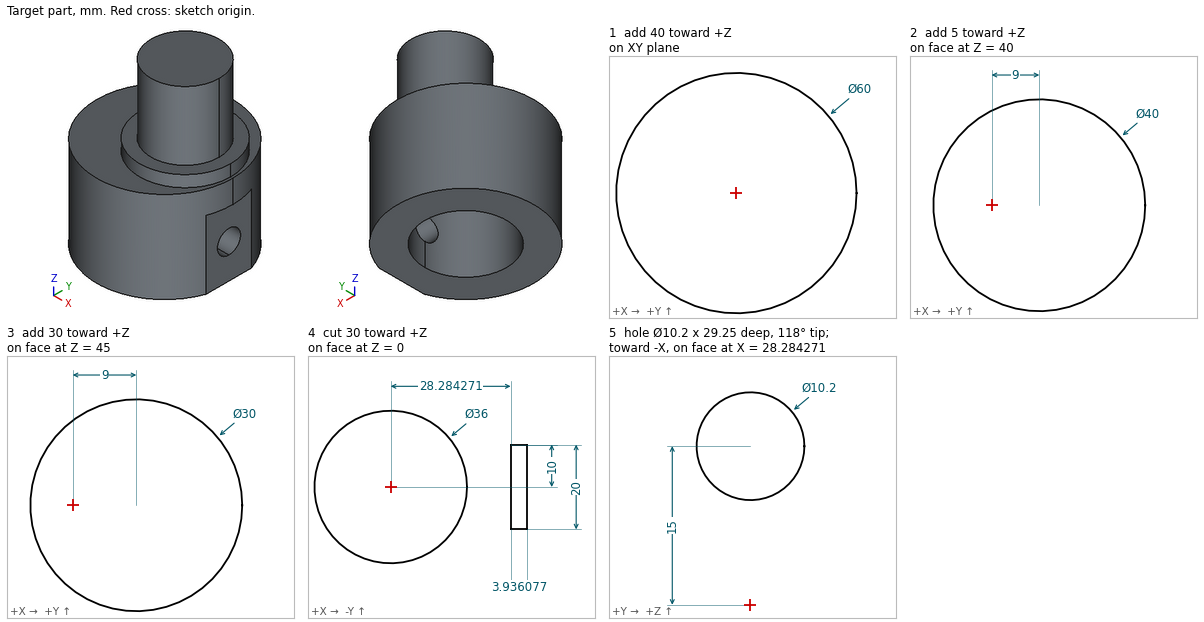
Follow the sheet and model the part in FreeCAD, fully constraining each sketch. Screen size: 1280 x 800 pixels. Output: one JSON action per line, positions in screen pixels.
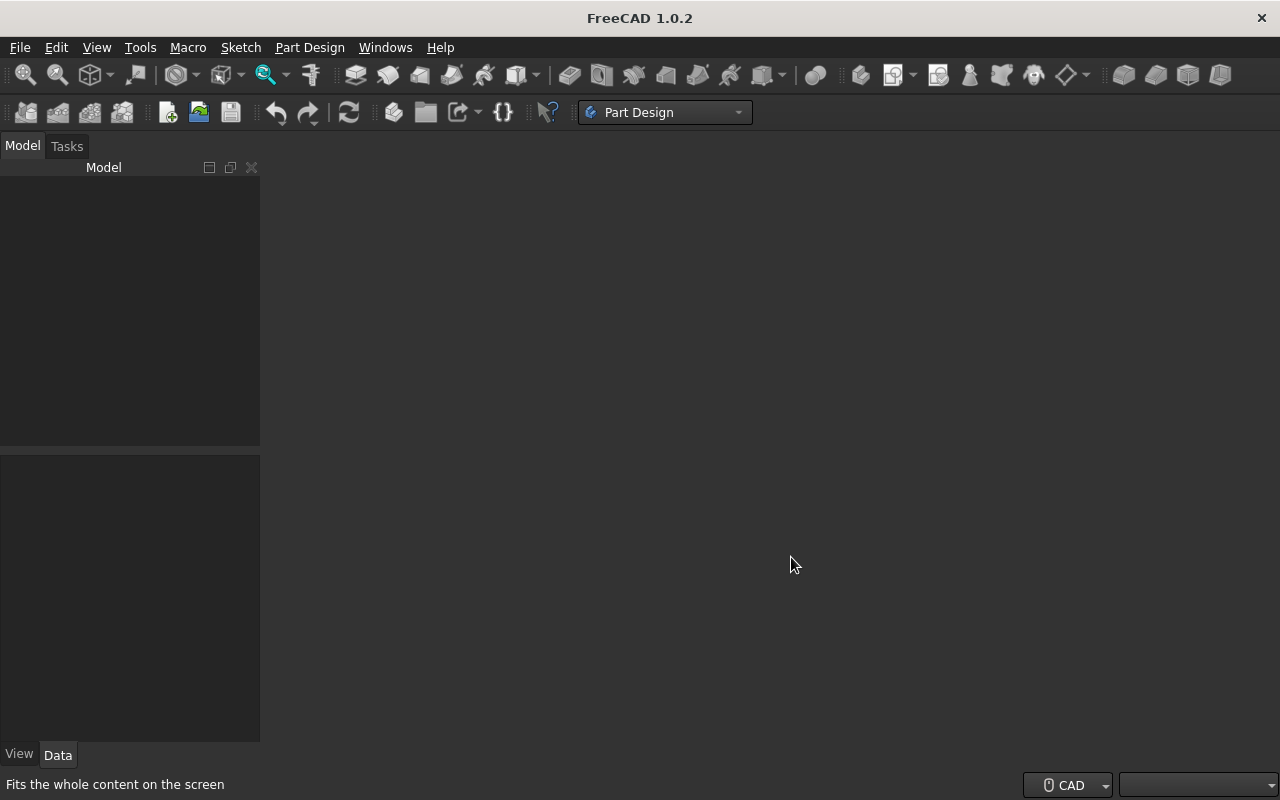
{"action": "key", "text": "ctrl+n"}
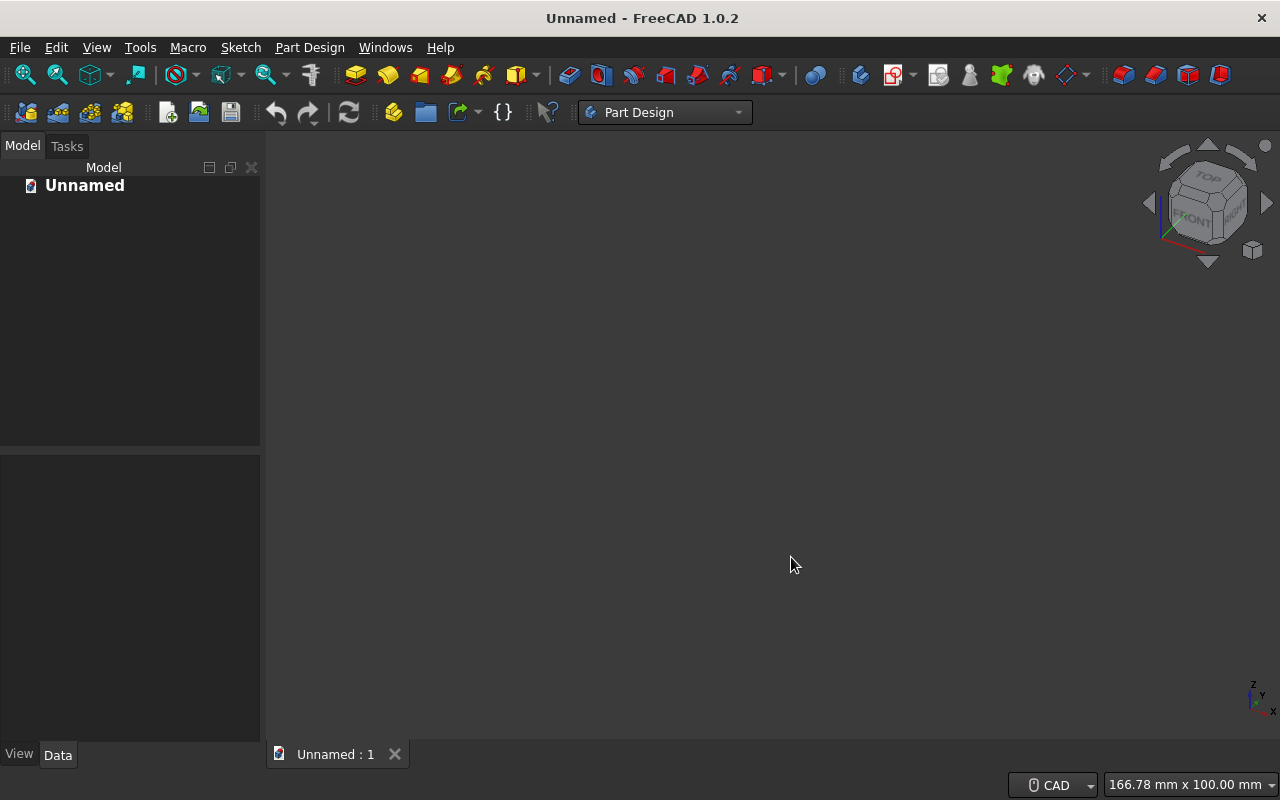
{"action": "left_click", "coordinate": [894, 76]}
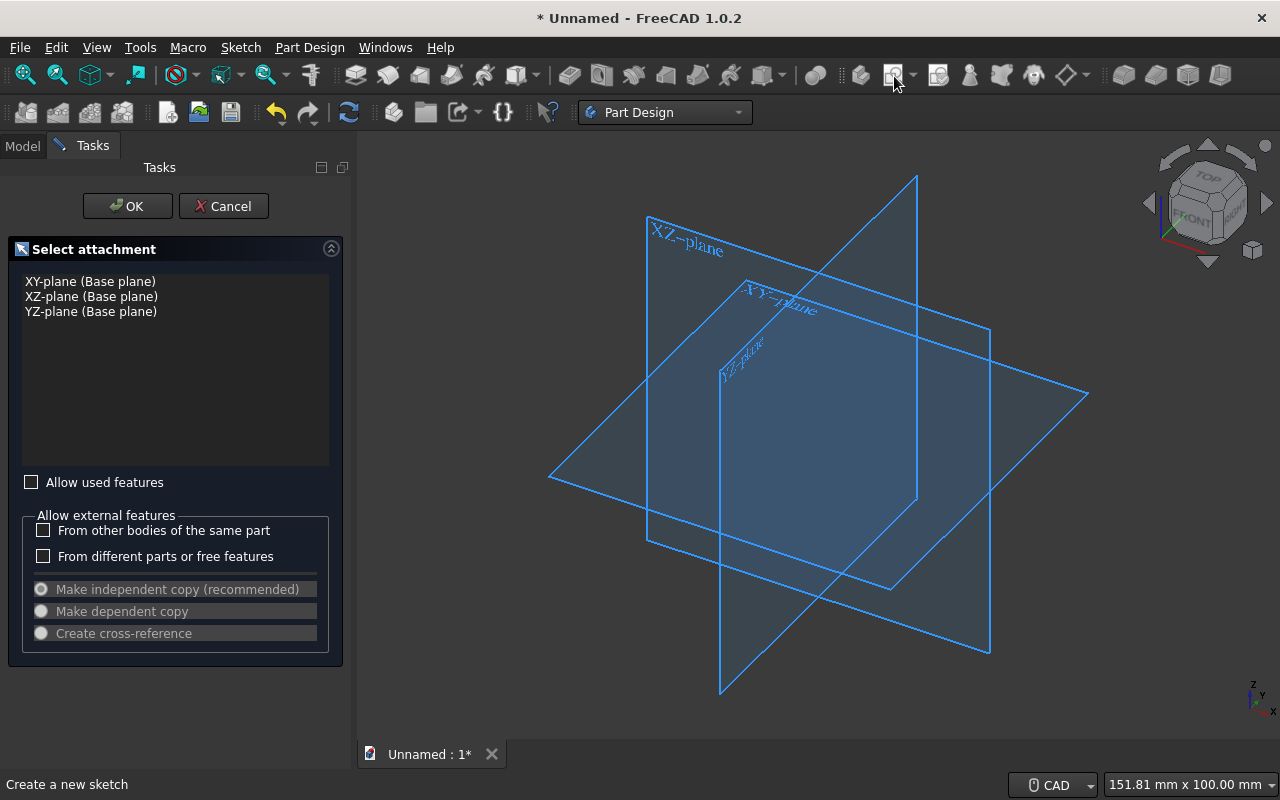
{"action": "left_click", "coordinate": [82, 282]}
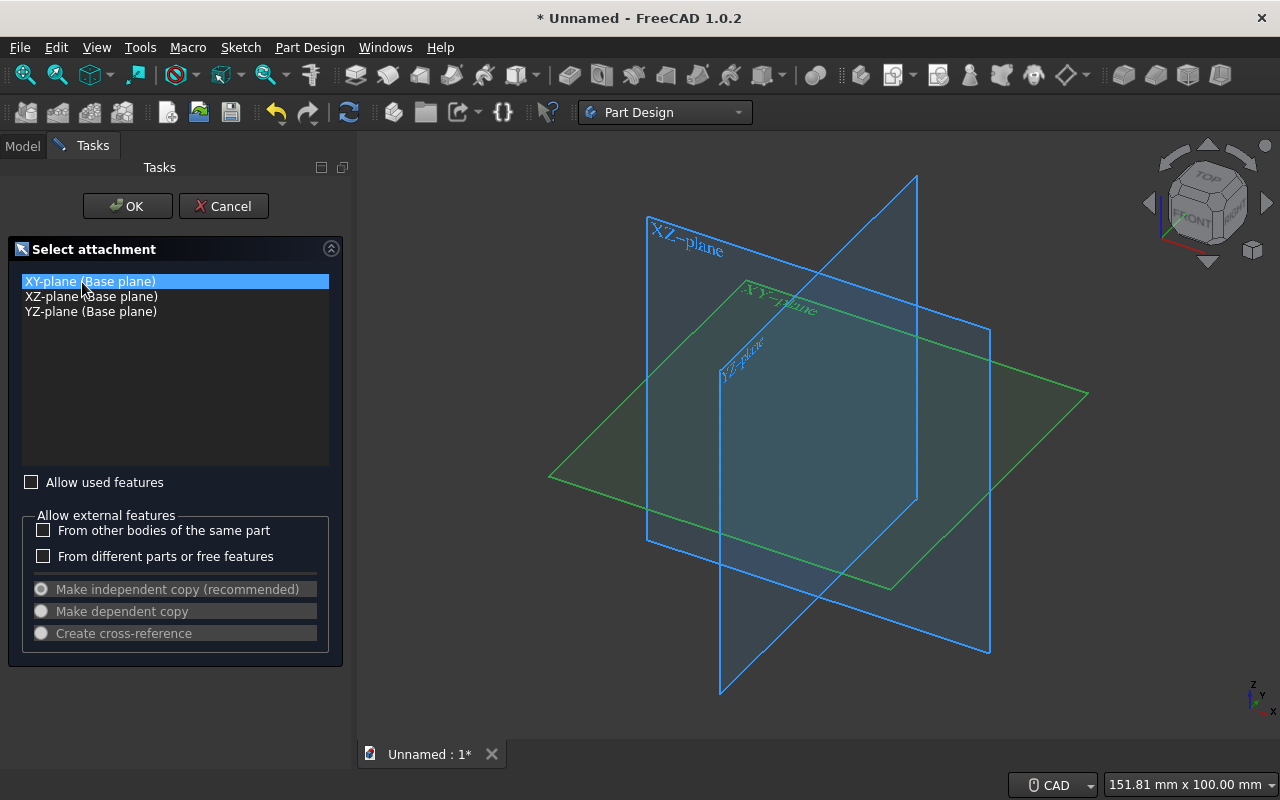
{"action": "left_click", "coordinate": [128, 206]}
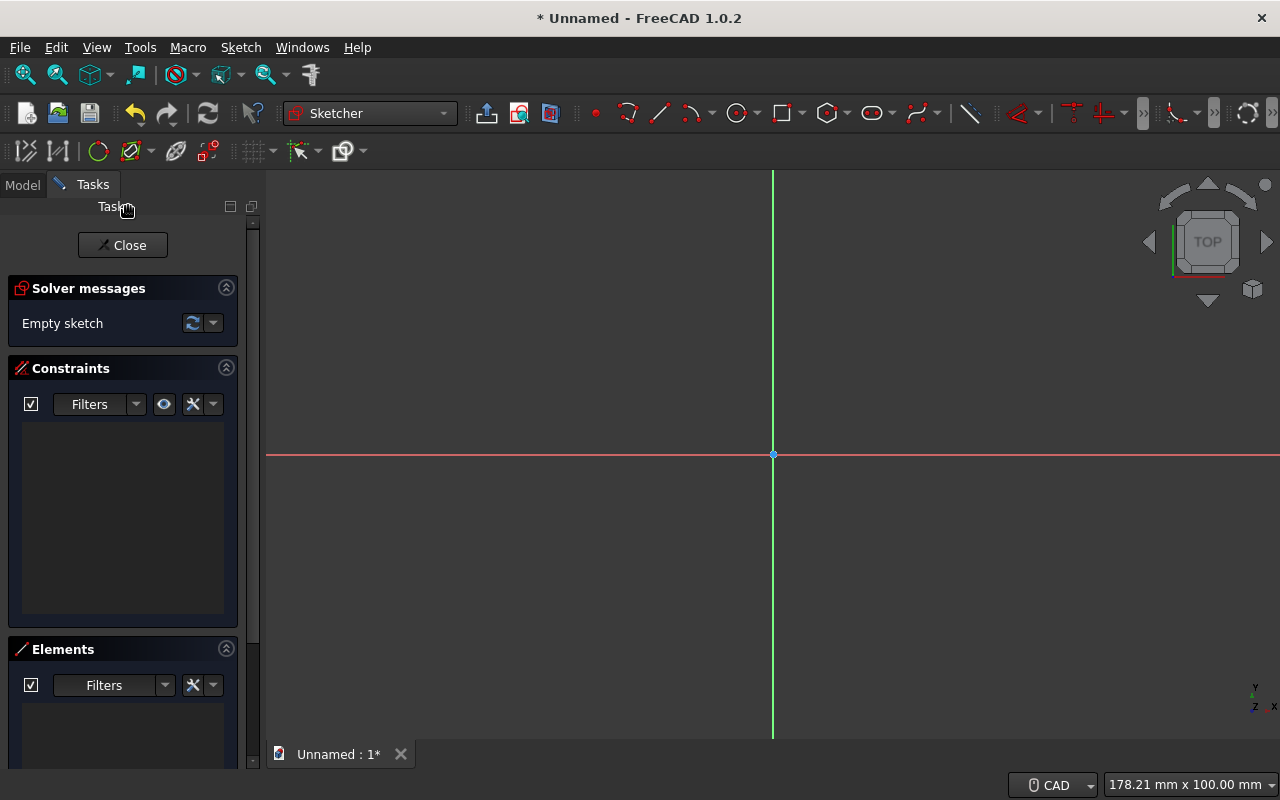
{"action": "left_click", "coordinate": [738, 114]}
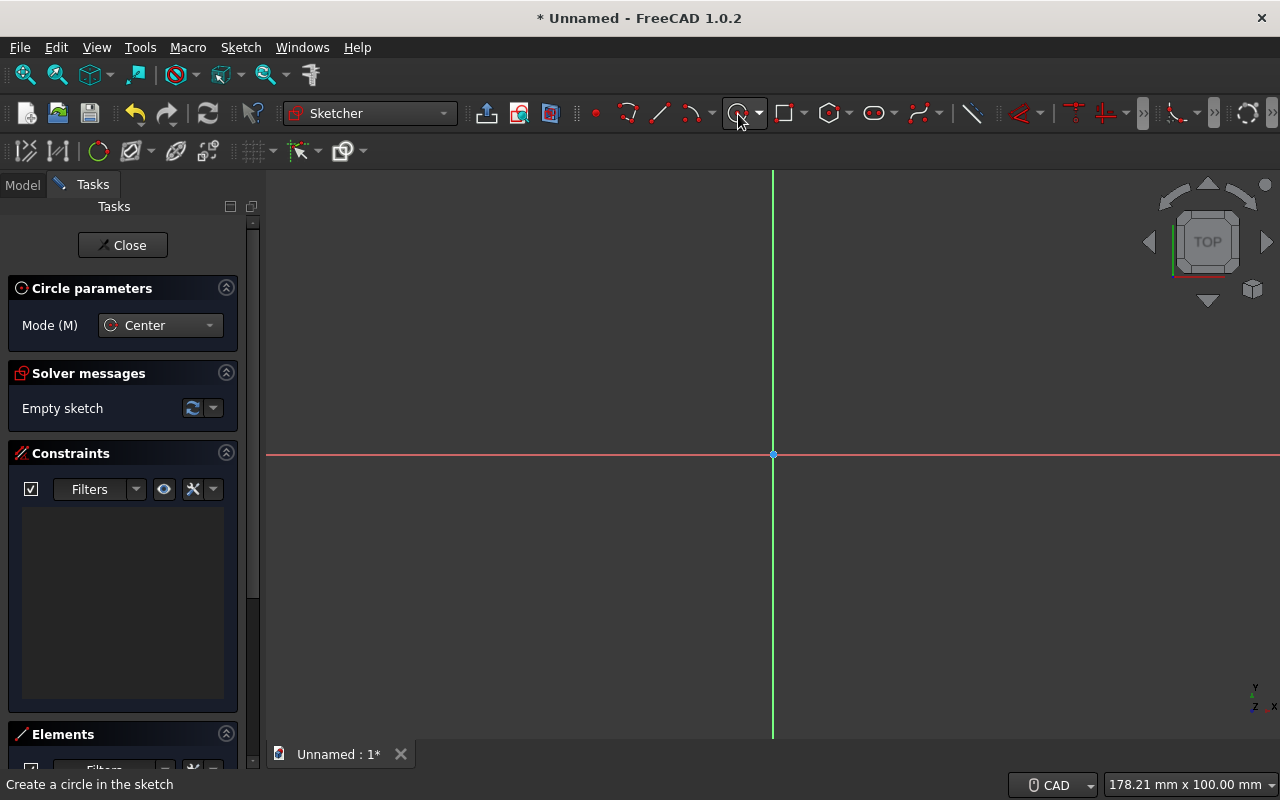
{"action": "left_click", "coordinate": [773, 454]}
{"action": "mouse_move", "coordinate": [894, 334]}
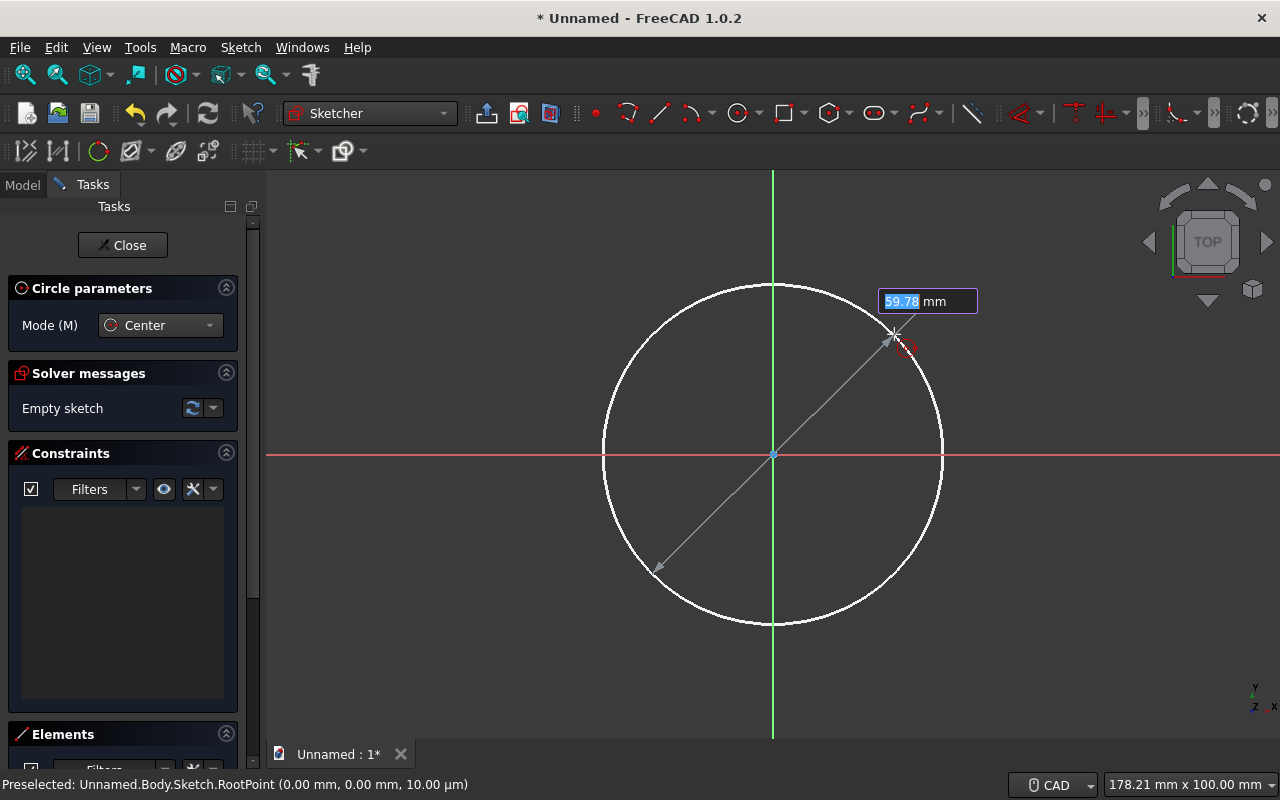
{"action": "type", "text": "60"}
{"action": "key", "text": "Return"}
{"action": "key", "text": "Escape"}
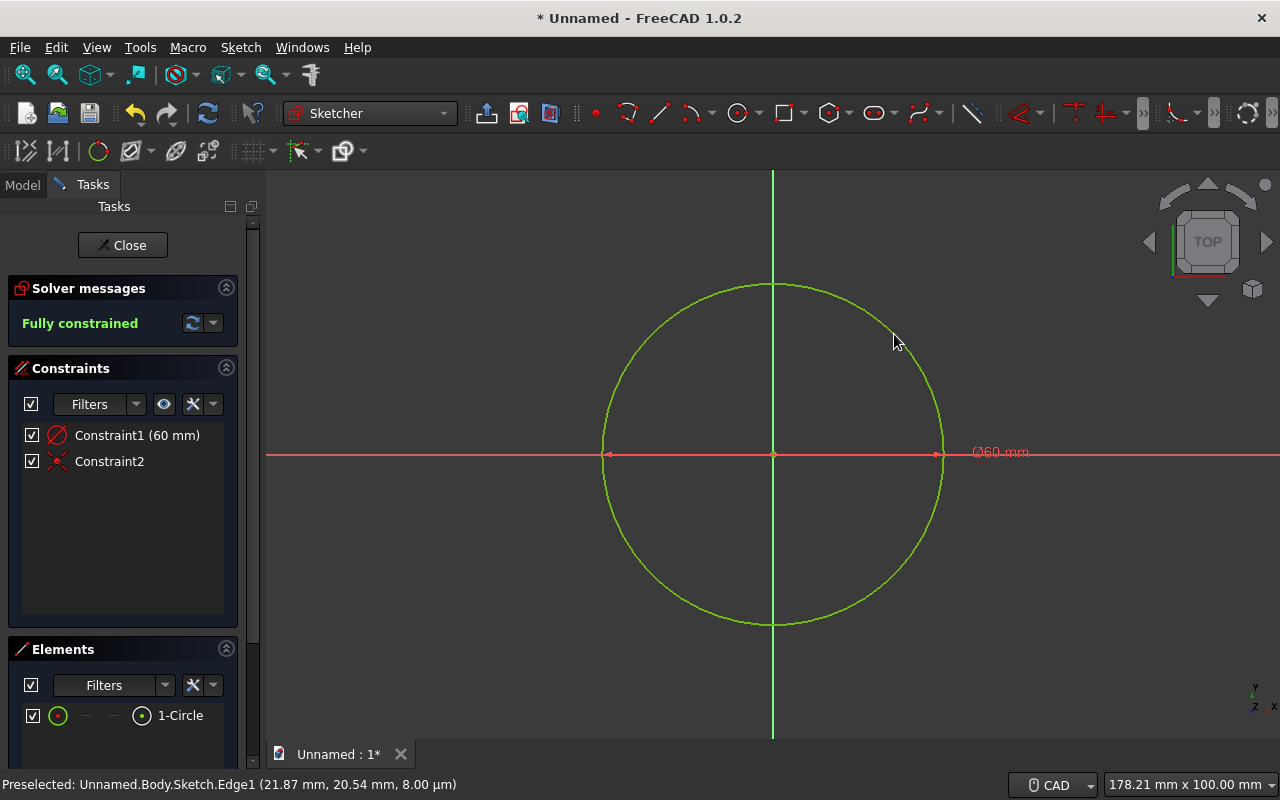
{"action": "left_click", "coordinate": [123, 245]}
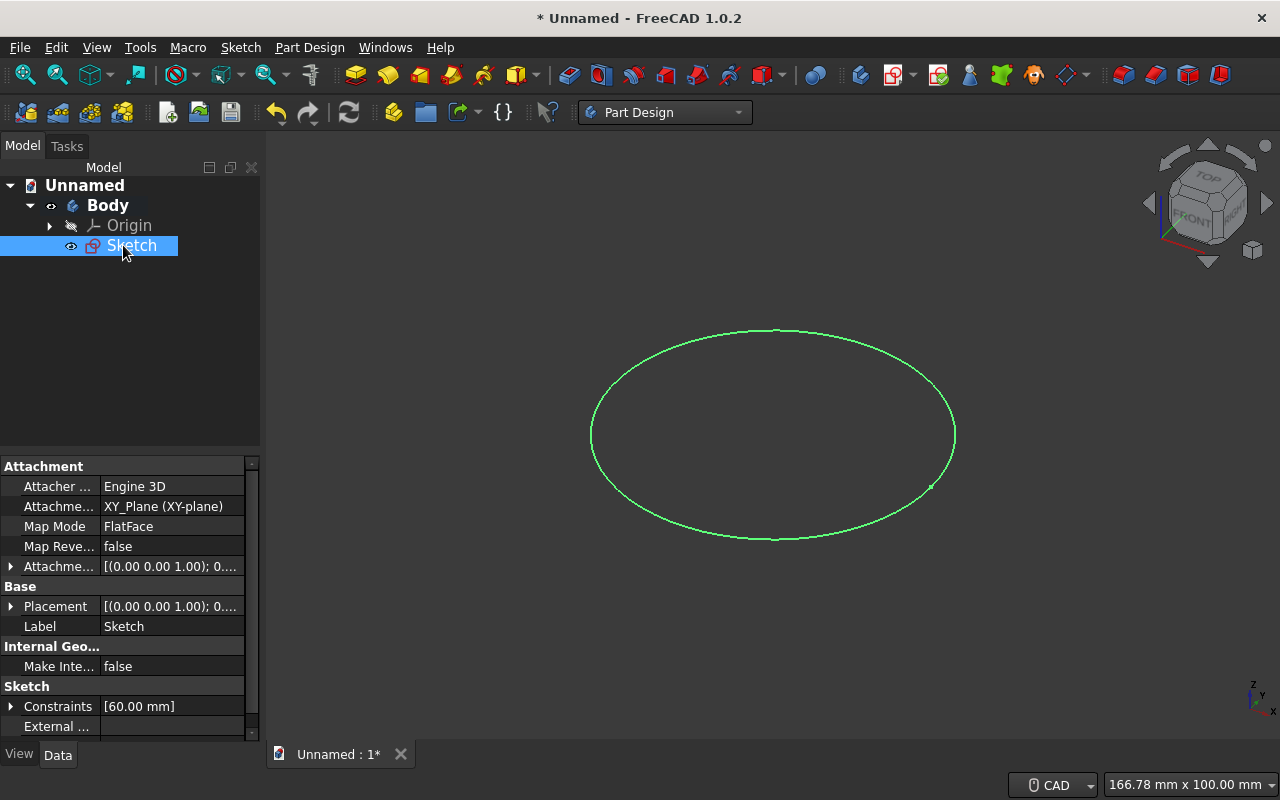
{"action": "left_click", "coordinate": [356, 76]}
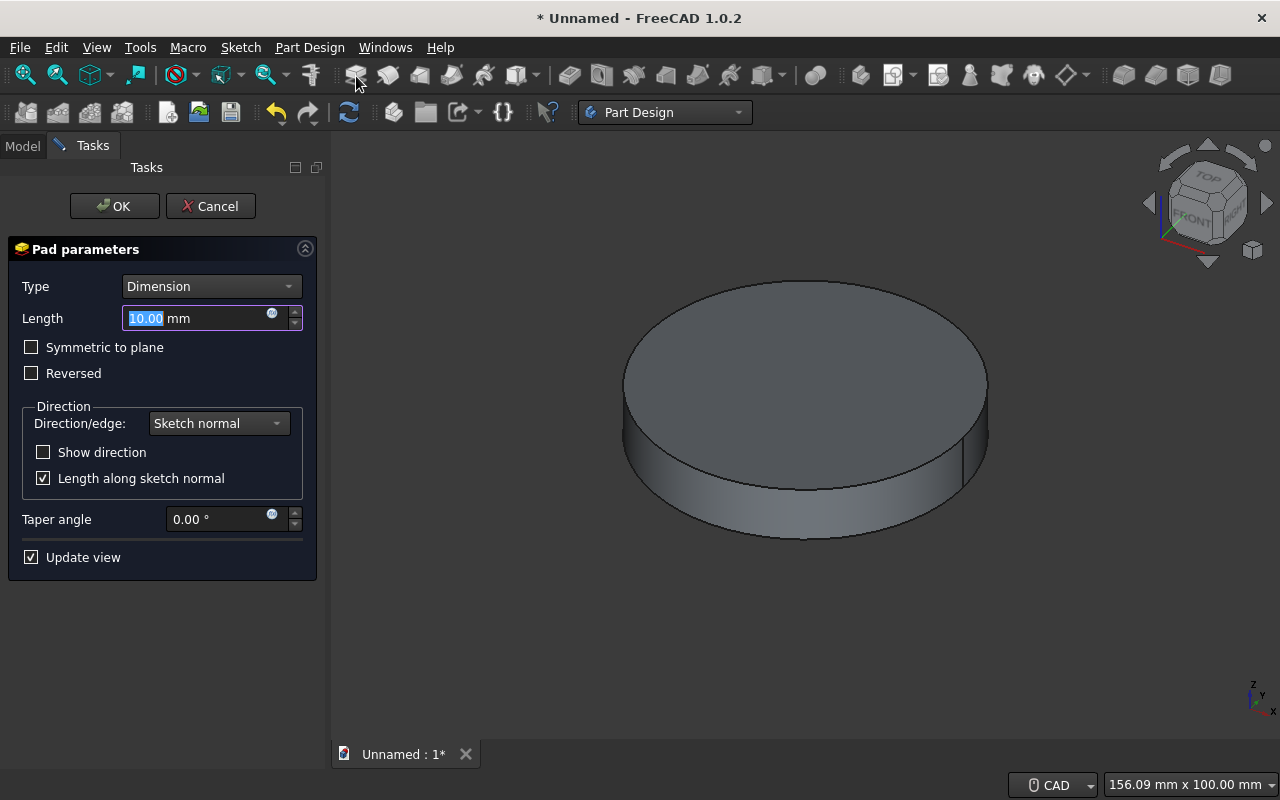
{"action": "type", "text": "40"}
{"action": "key", "text": "Tab"}